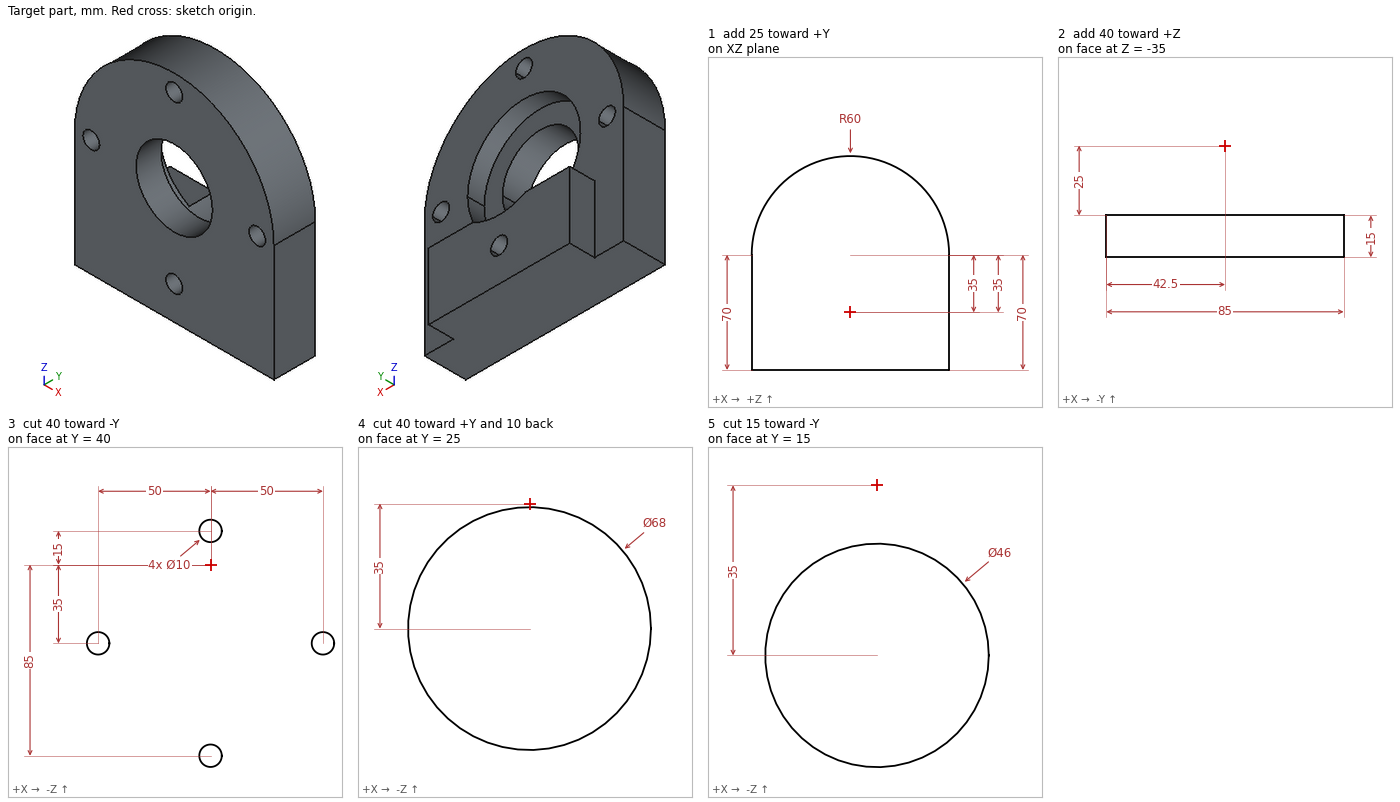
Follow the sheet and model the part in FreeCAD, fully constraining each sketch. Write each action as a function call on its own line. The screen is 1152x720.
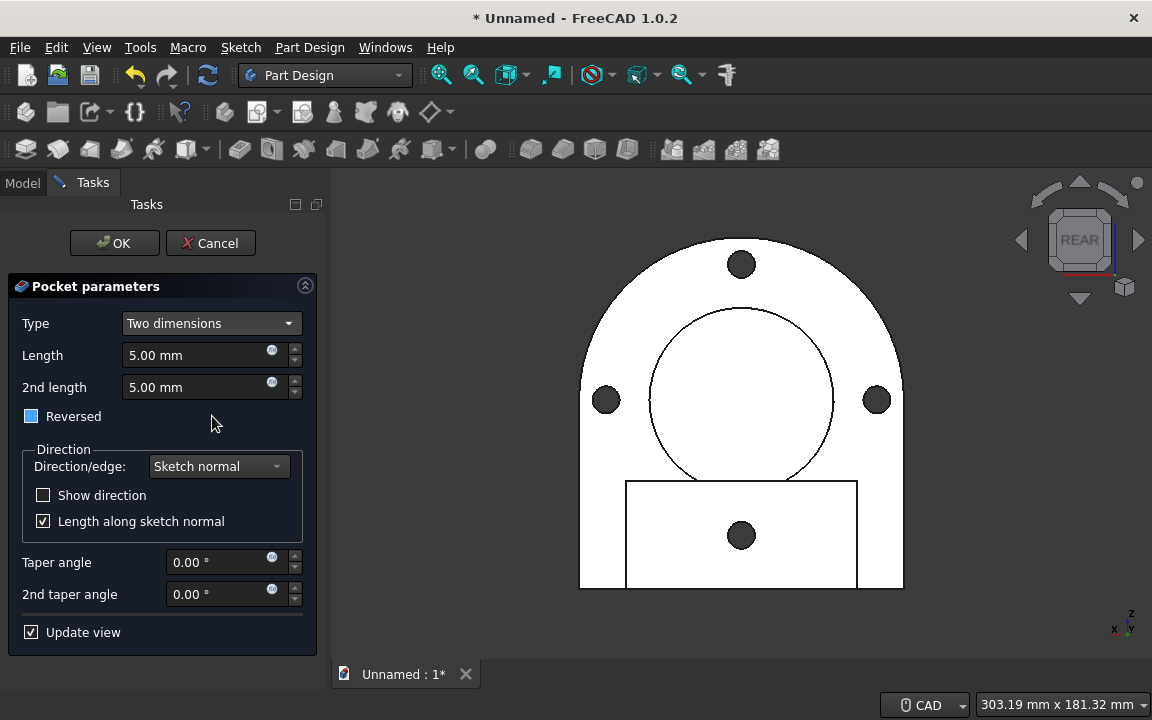
triple_click(204, 355)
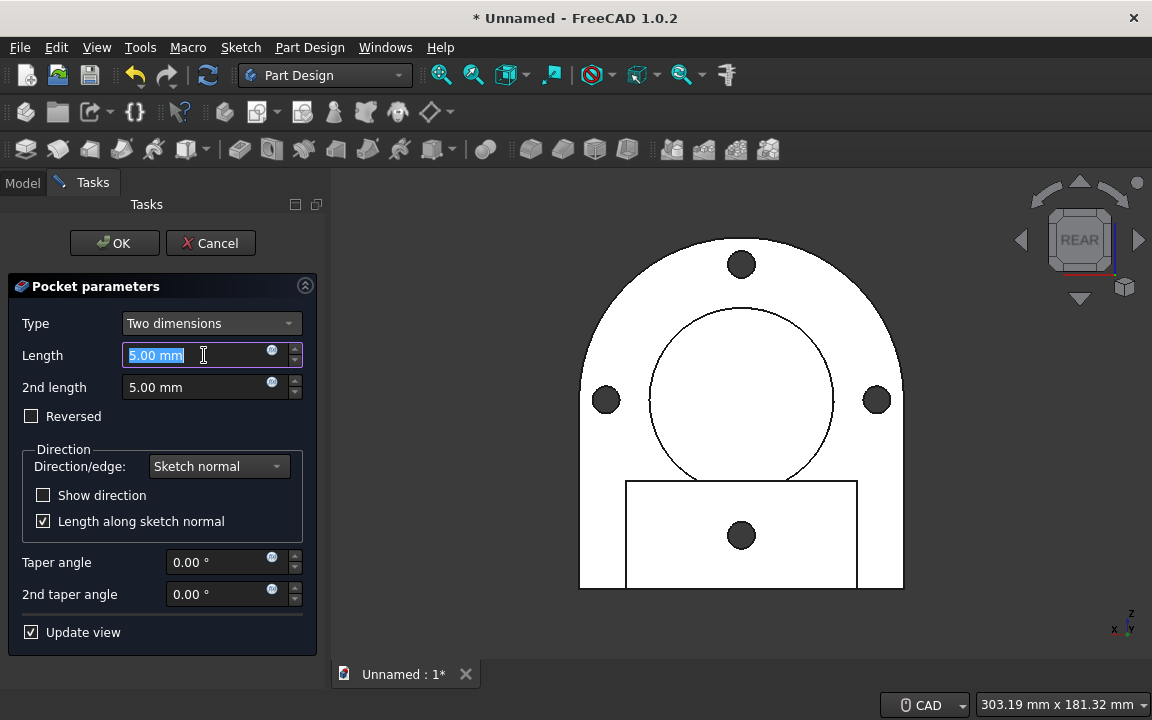
text(40)
key(Tab)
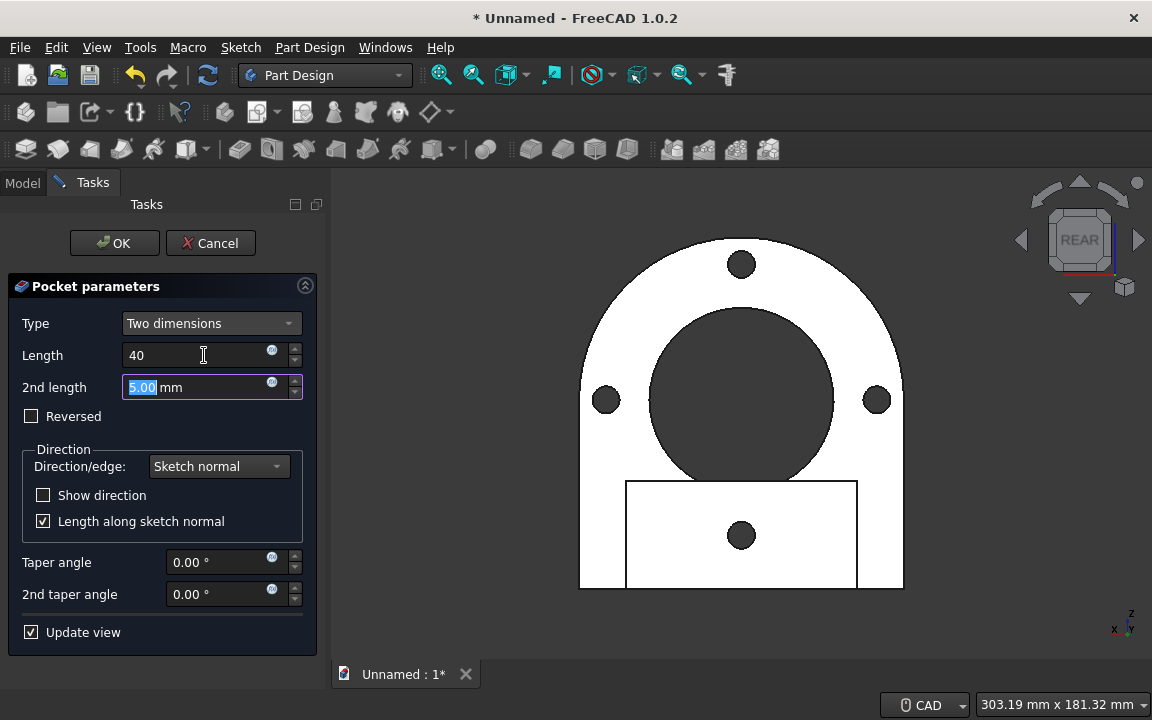
text(10)
key(Tab)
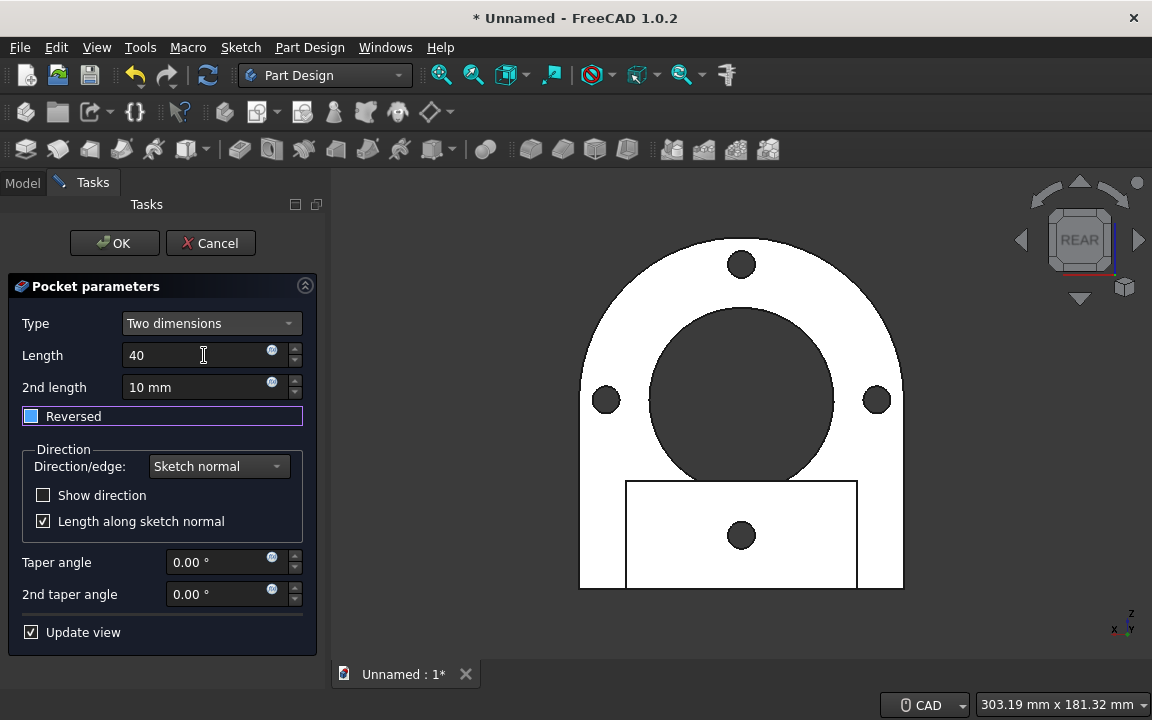
click(30, 416)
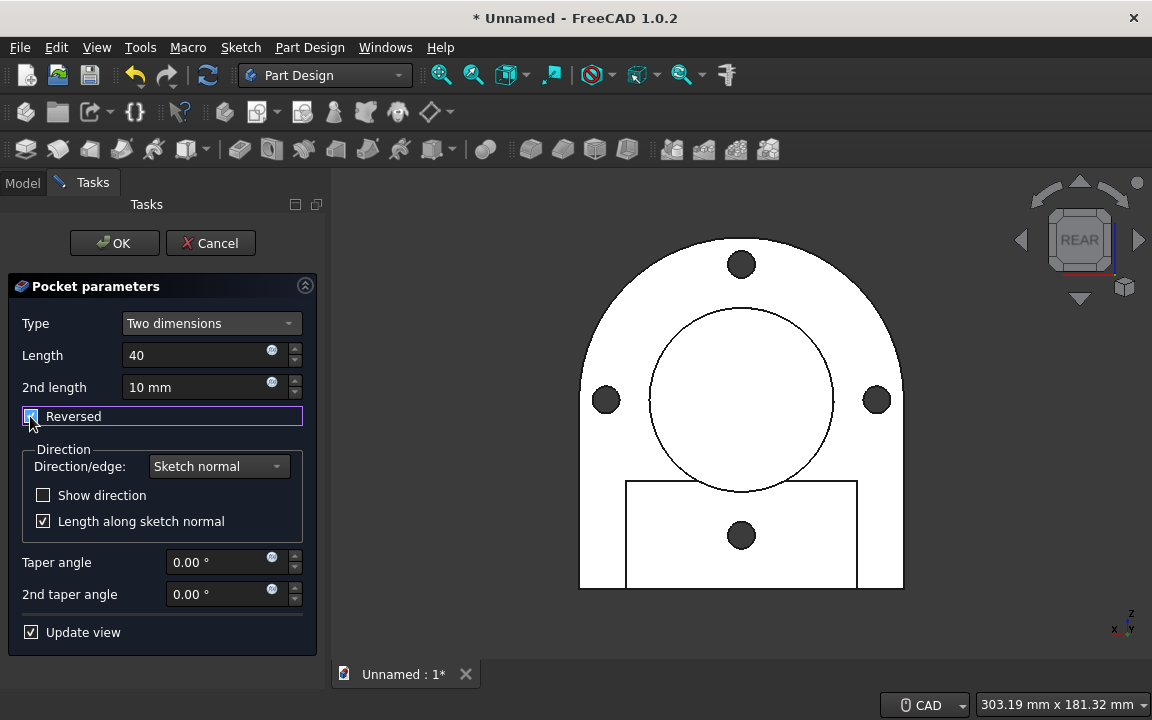
click(115, 243)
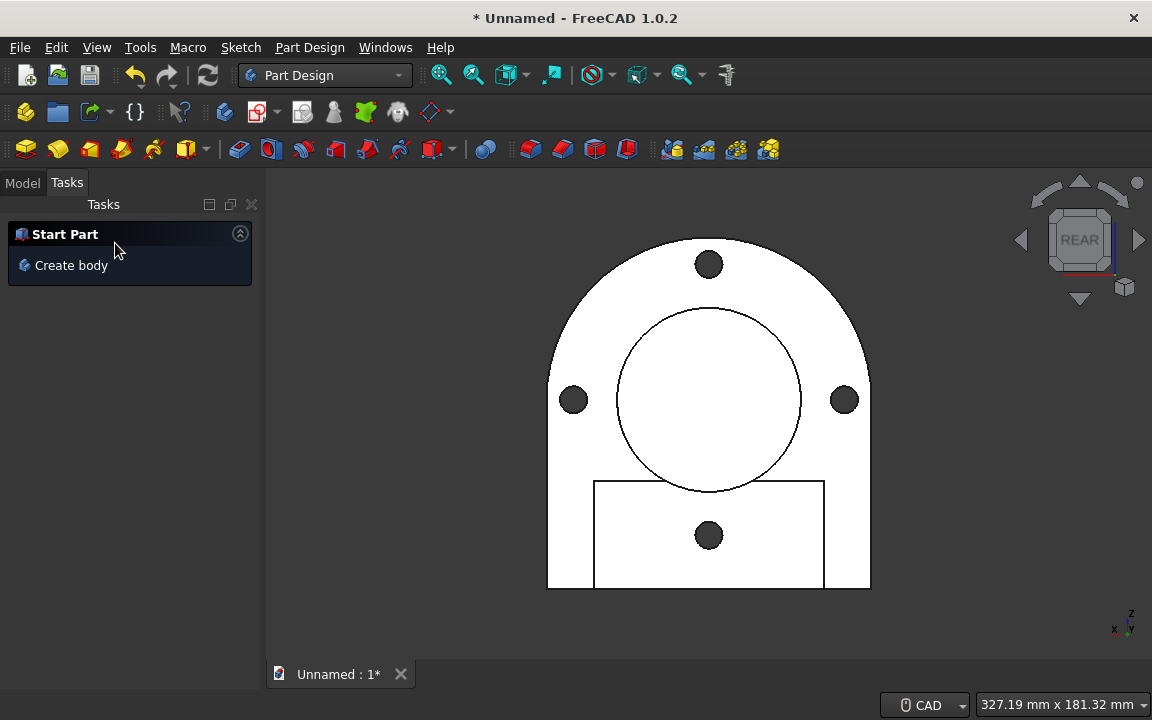
click(709, 399)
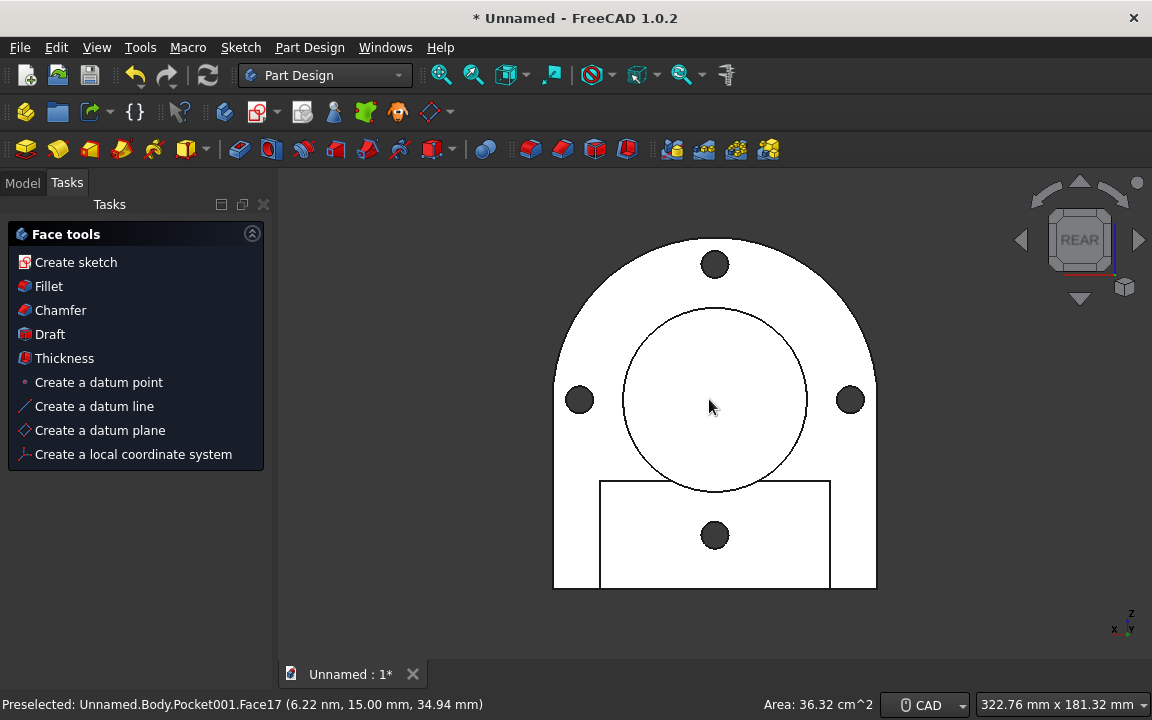
click(258, 112)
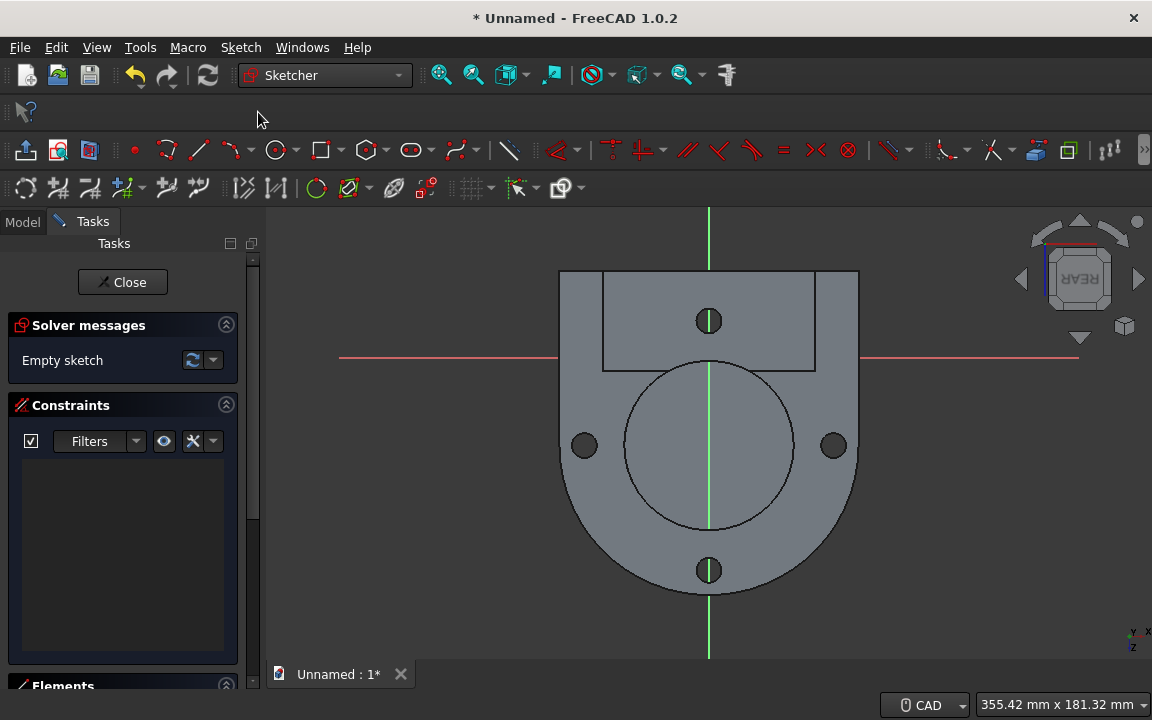
key(q)
key(s)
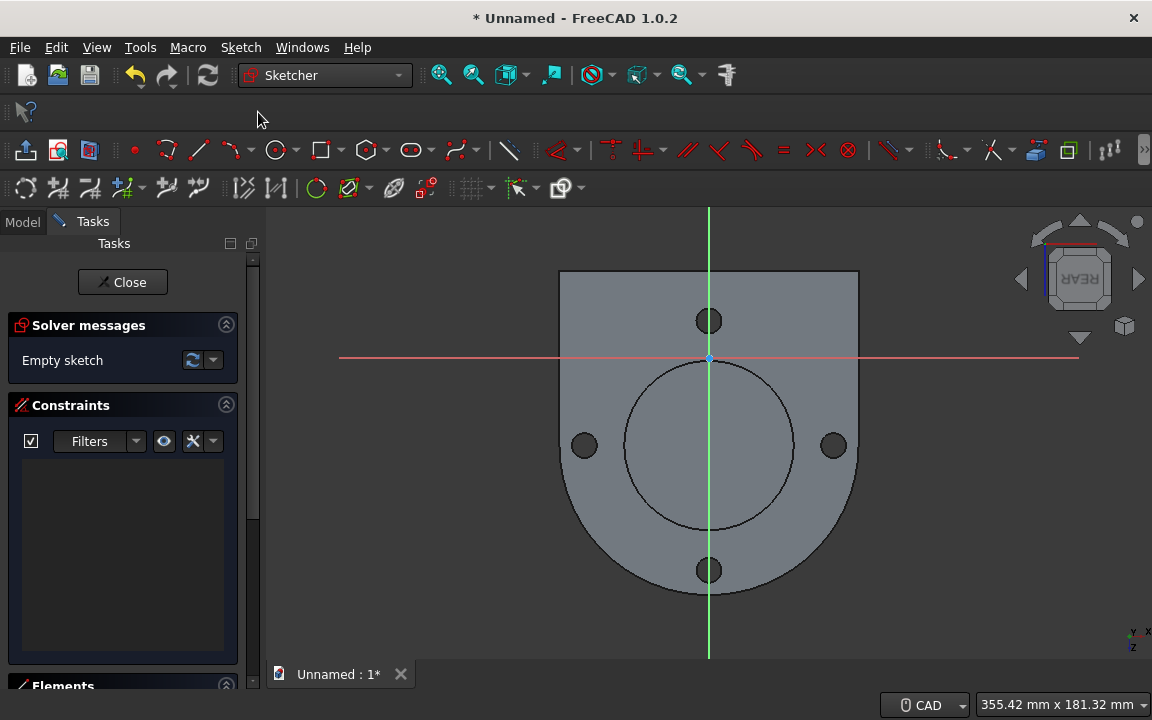
scroll(792, 428, up, 3)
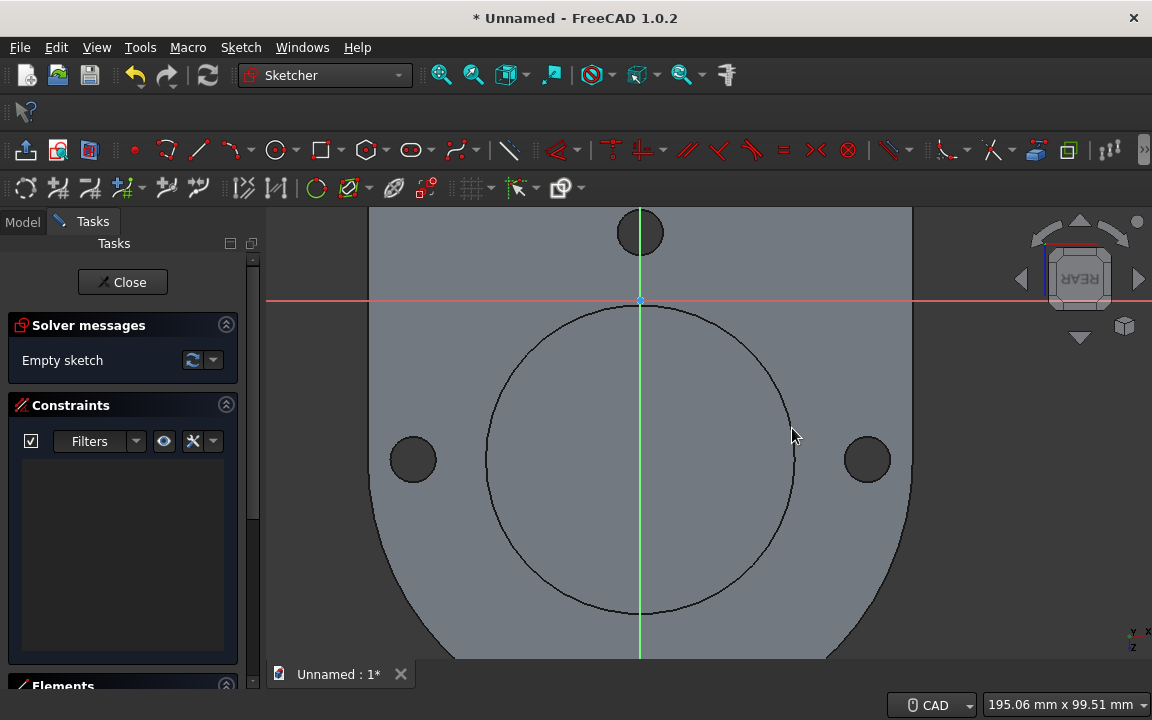
key(g)
key(c)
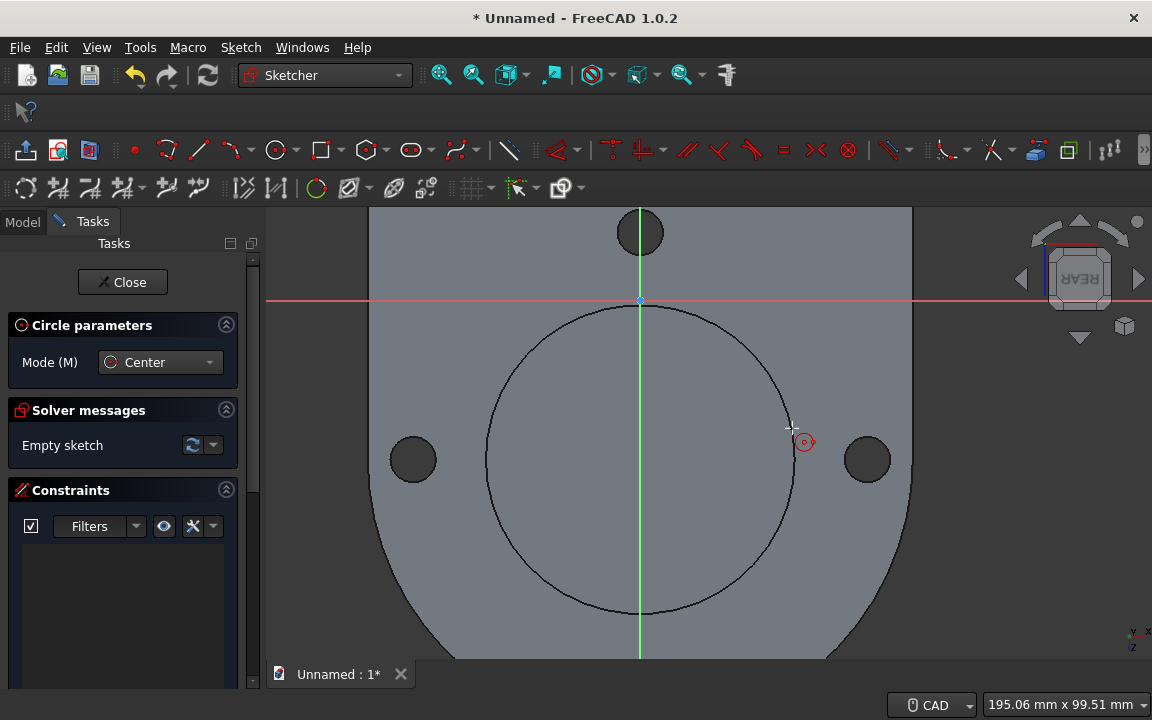
click(640, 460)
move(714, 386)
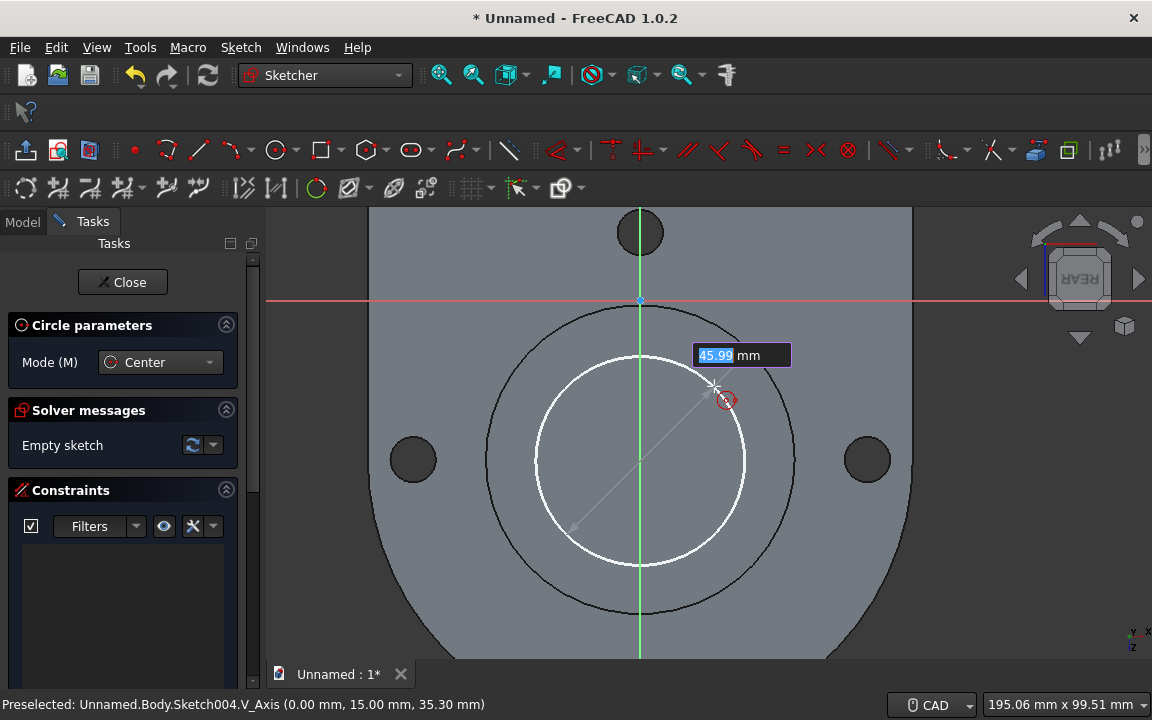
text(46)
key(Return)
key(Escape)